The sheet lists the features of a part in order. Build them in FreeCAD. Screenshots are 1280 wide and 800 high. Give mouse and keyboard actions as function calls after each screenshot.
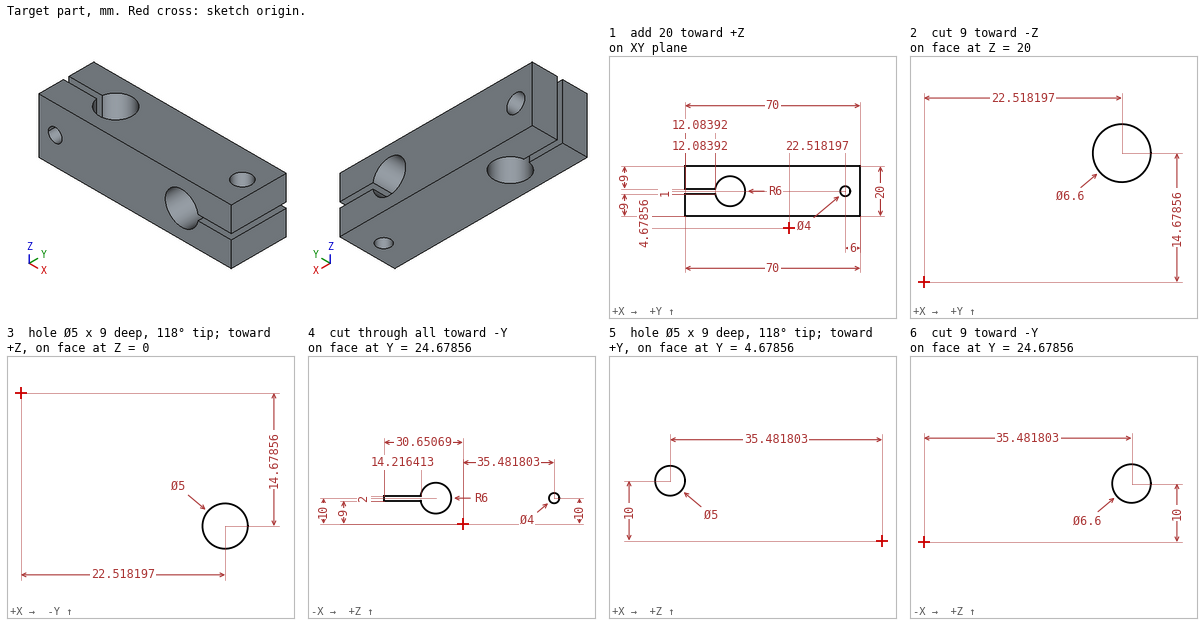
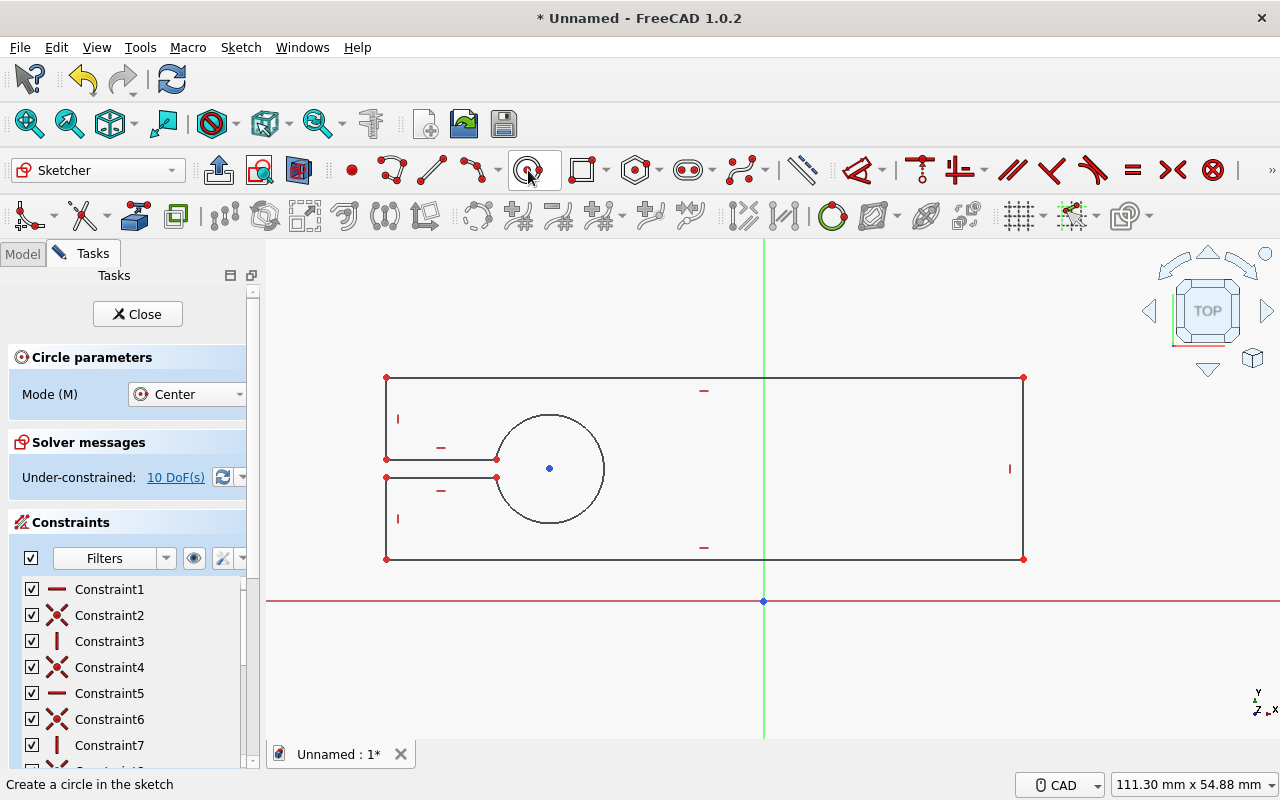
scroll(969, 468, up, 2)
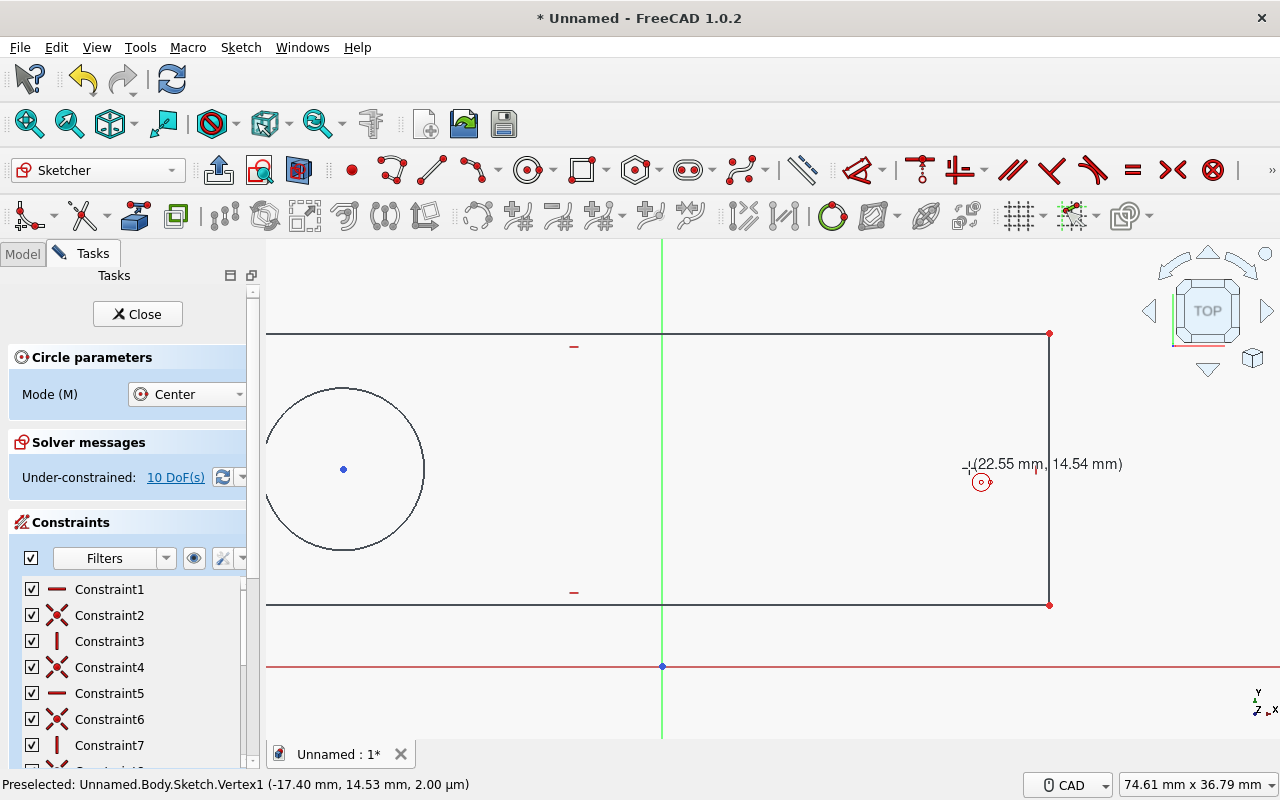
click(968, 467)
click(987, 448)
key(Escape)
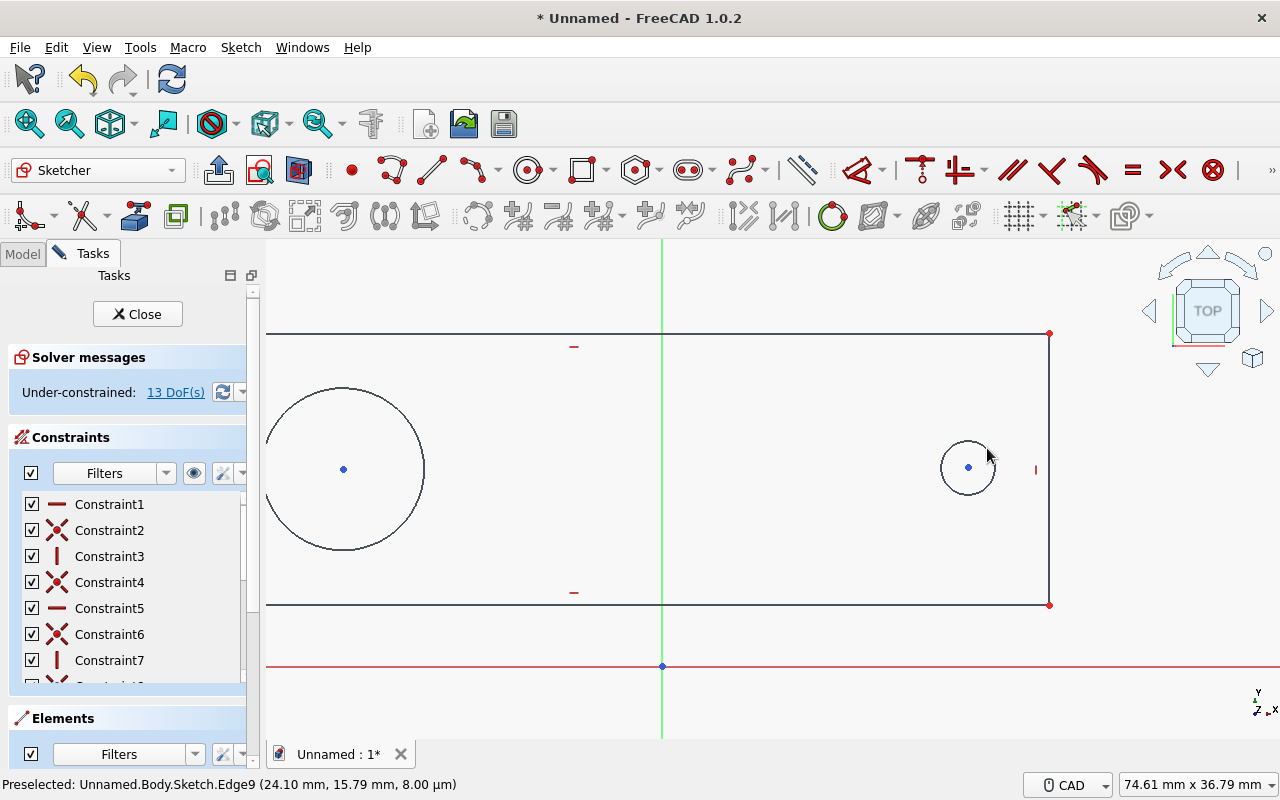
click(858, 170)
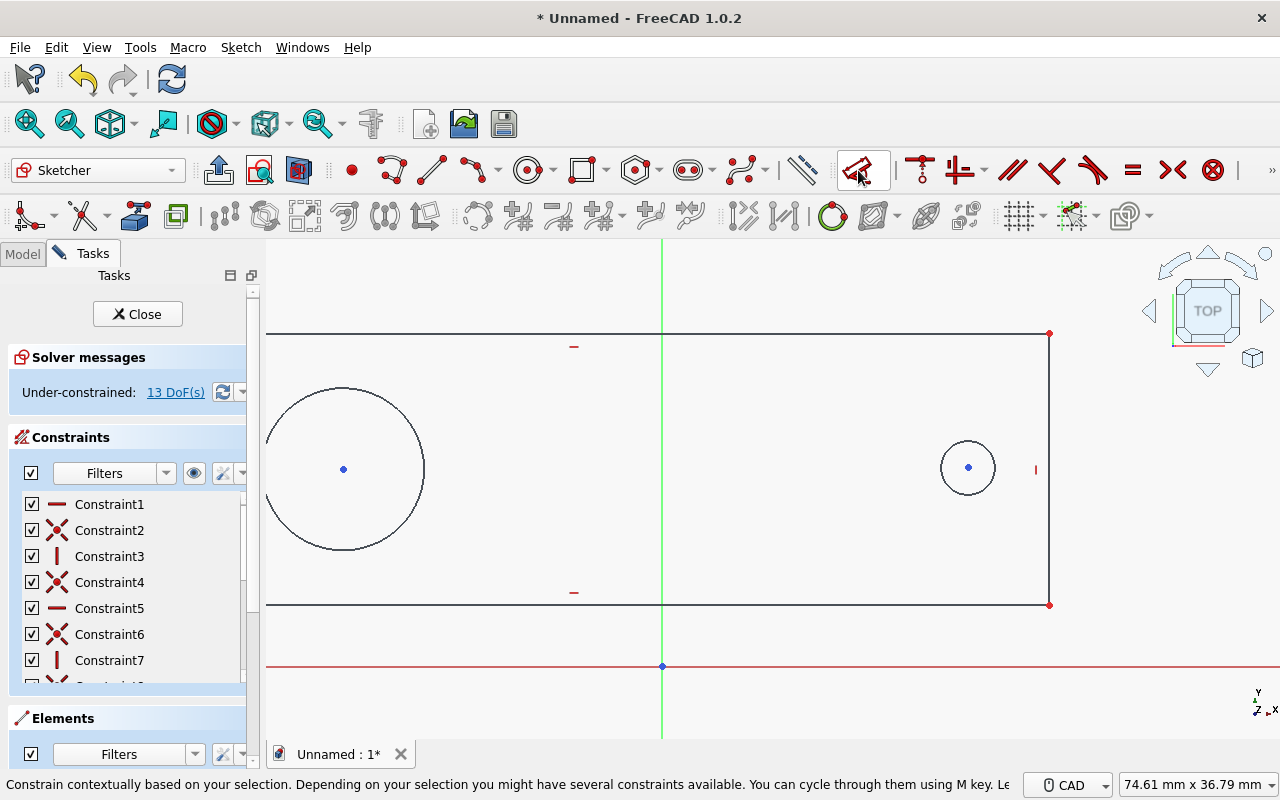
click(373, 545)
click(385, 575)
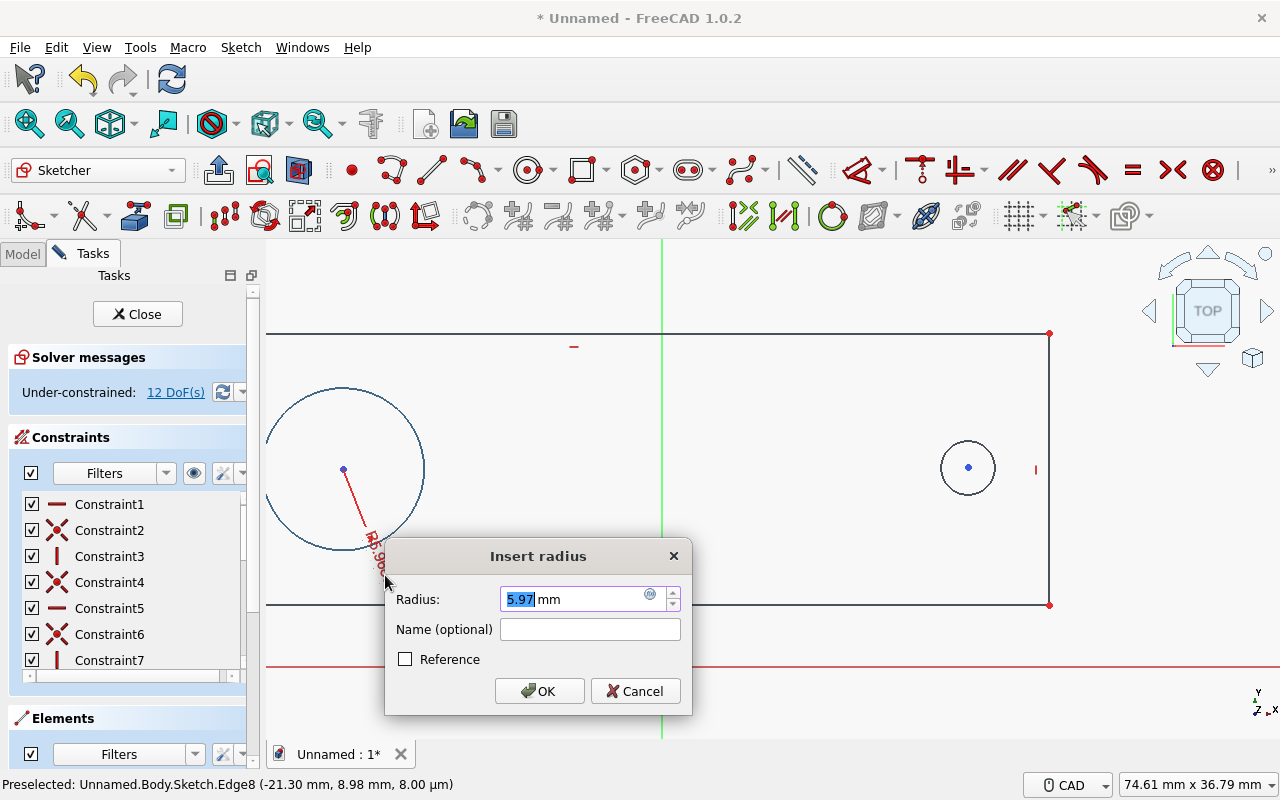
text(6)
key(Return)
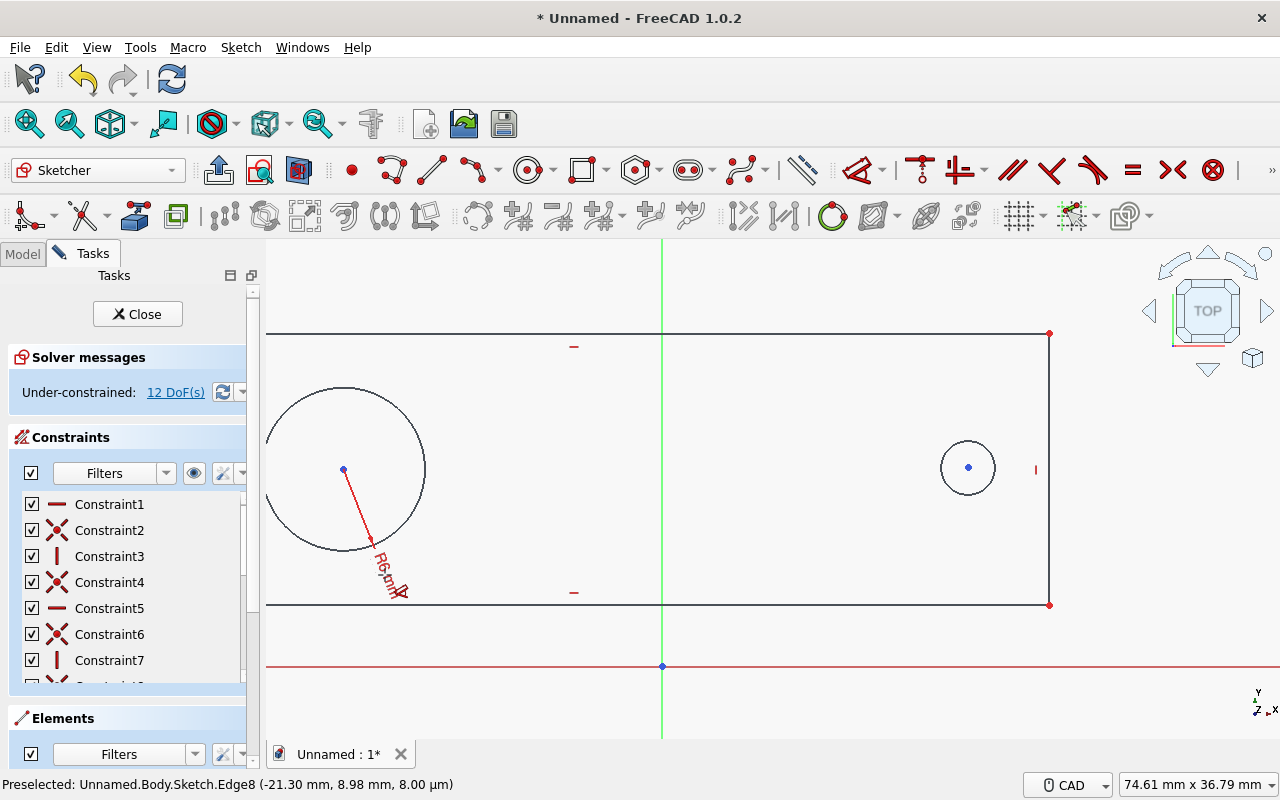
click(987, 449)
click(1010, 426)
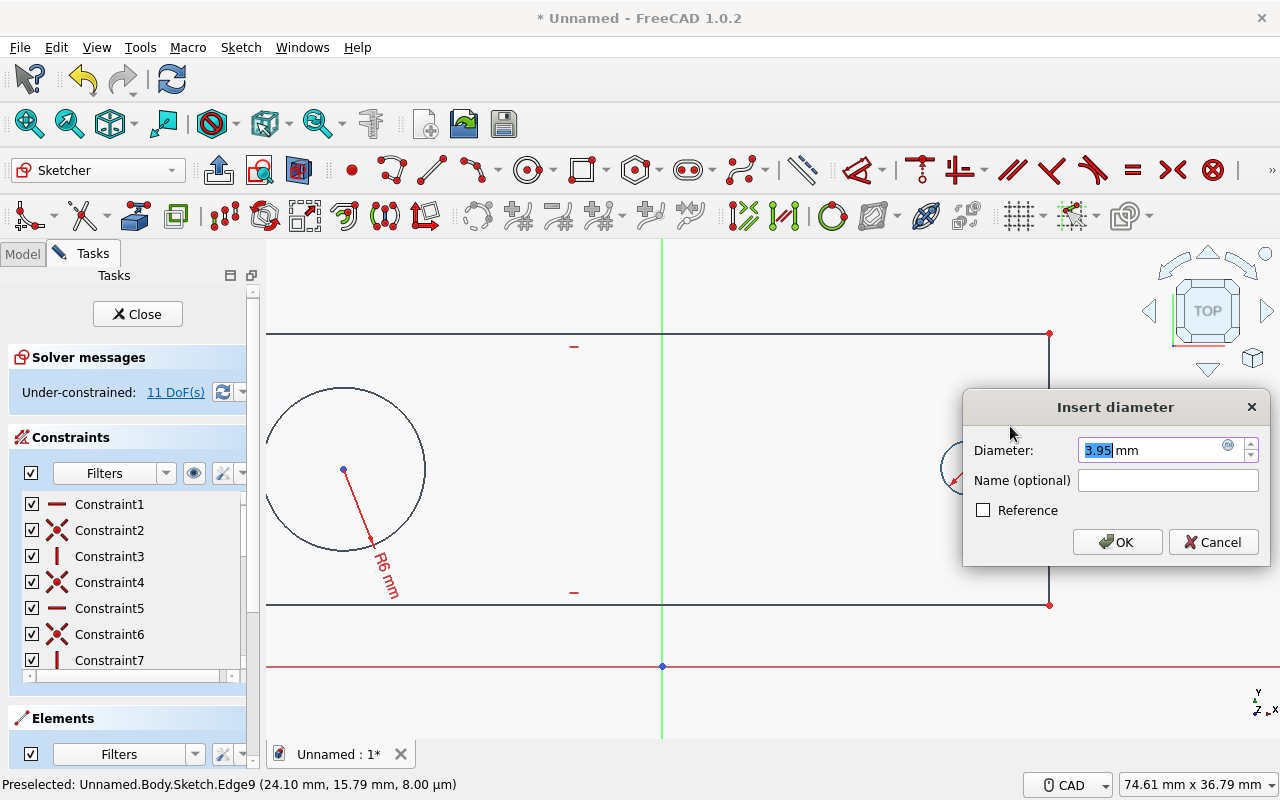
text(4)
key(Return)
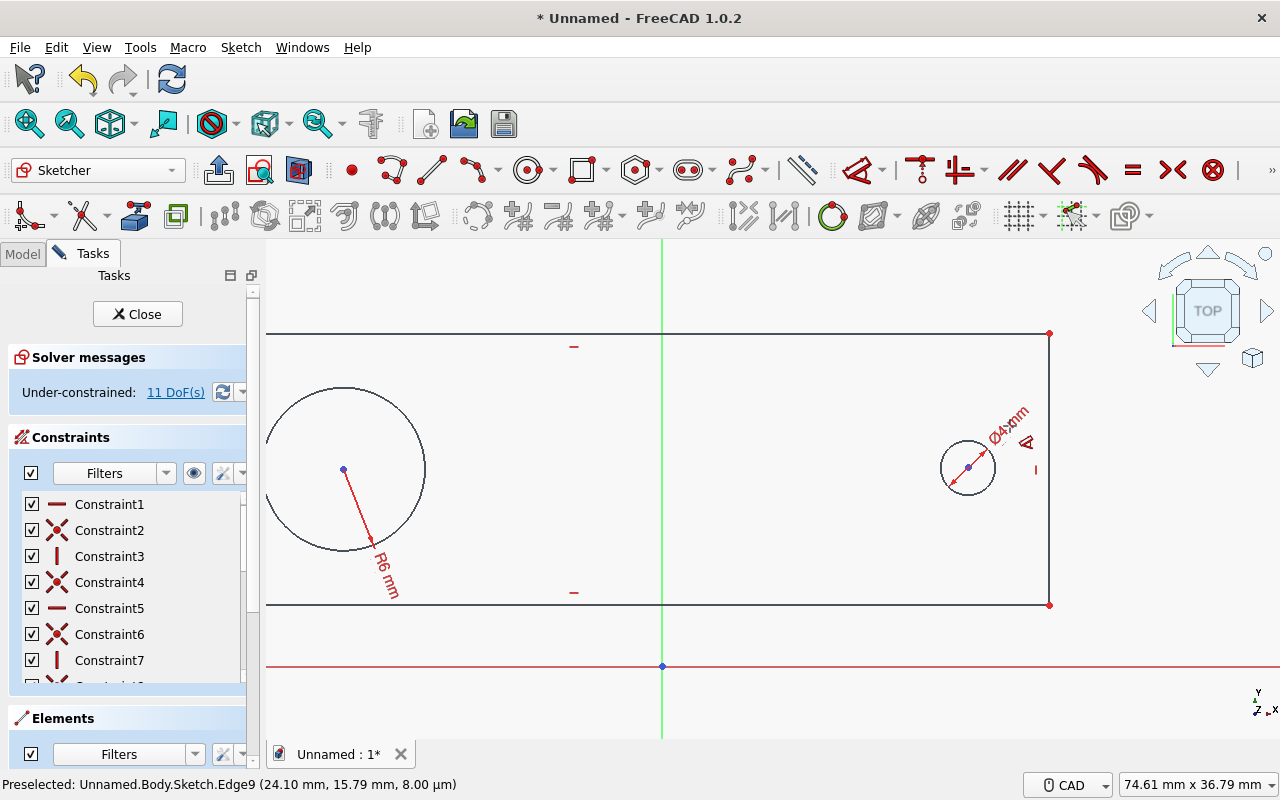
scroll(970, 468, down, 2)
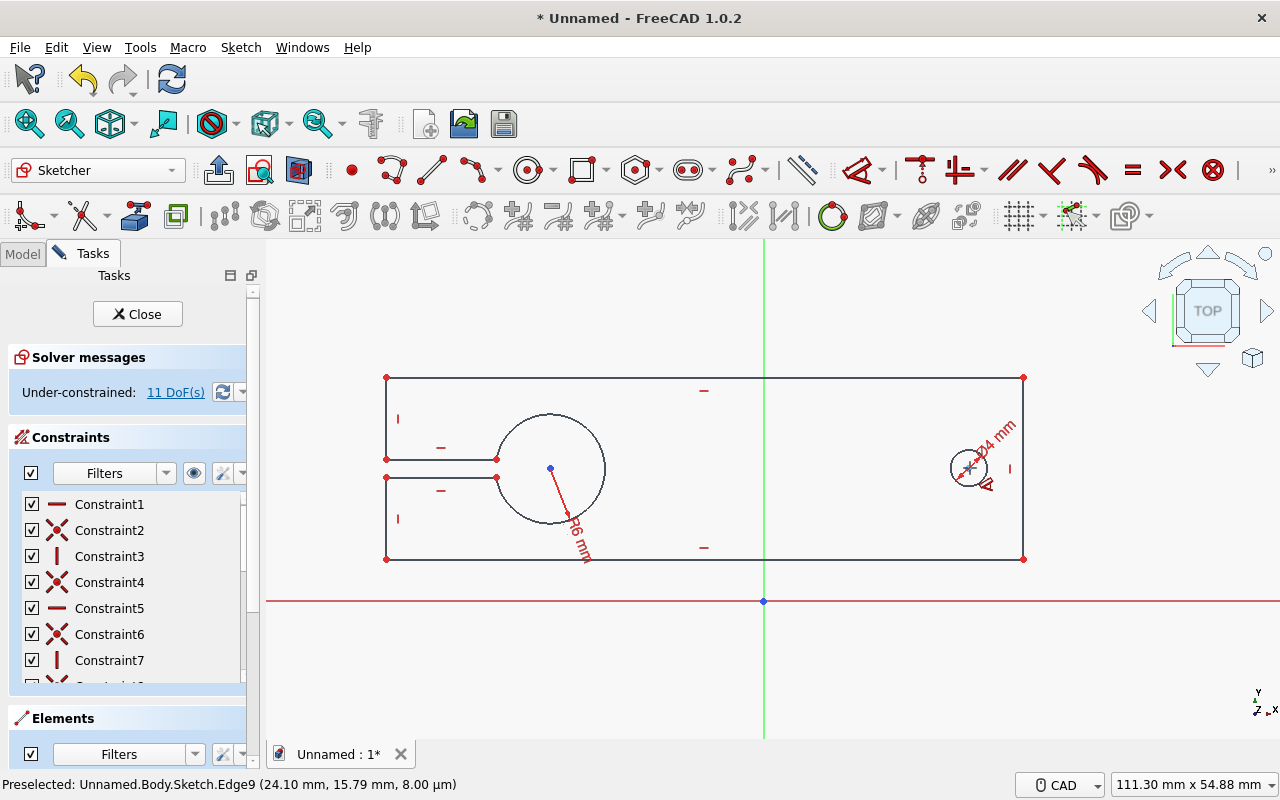
click(386, 503)
click(352, 519)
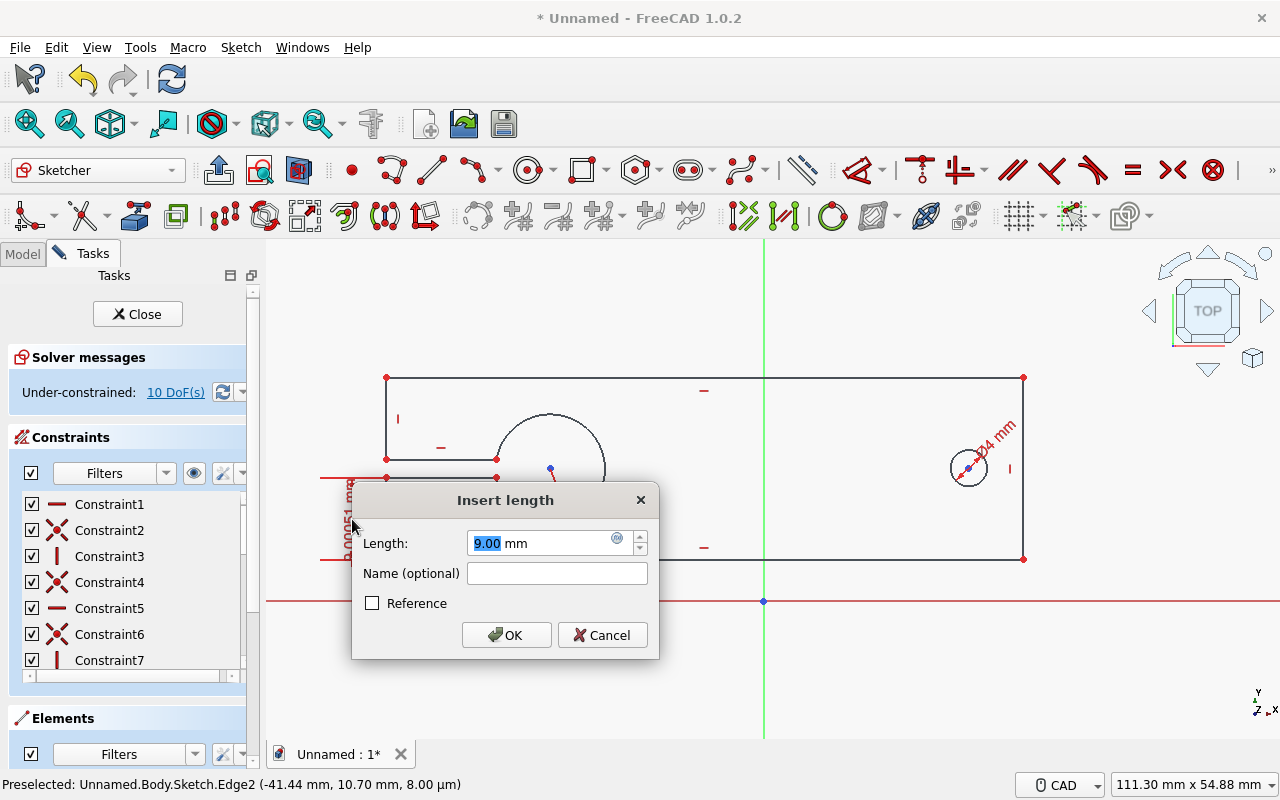
text(9)
key(Return)